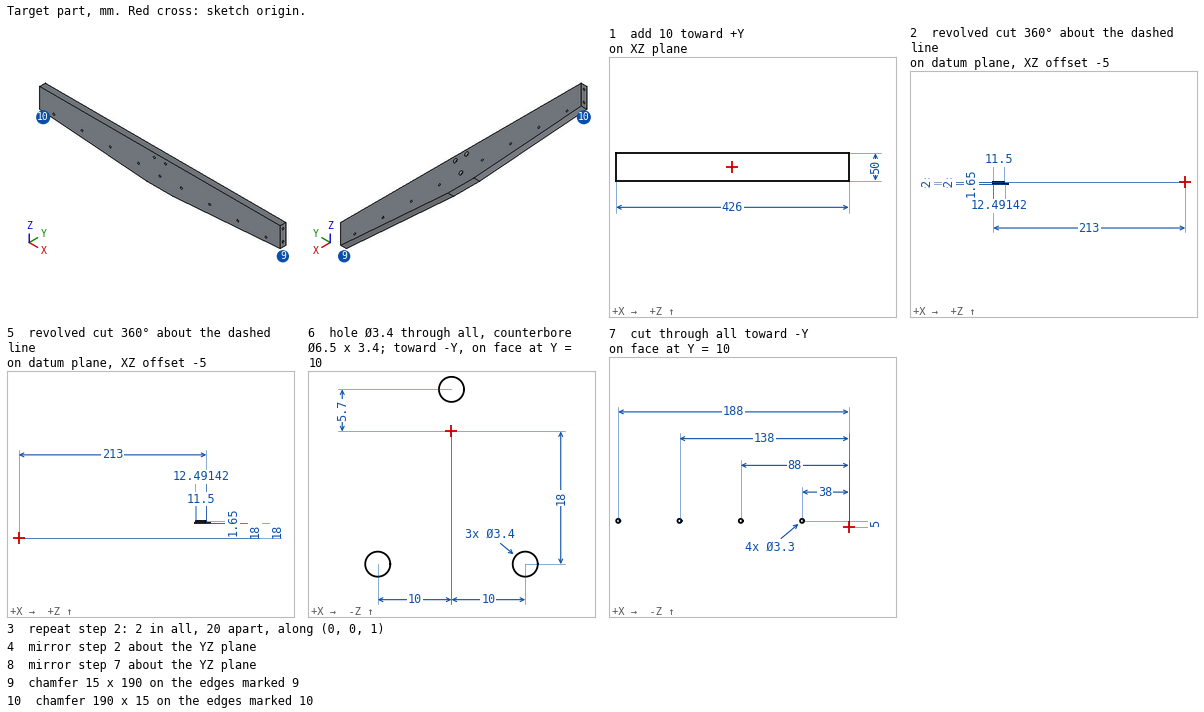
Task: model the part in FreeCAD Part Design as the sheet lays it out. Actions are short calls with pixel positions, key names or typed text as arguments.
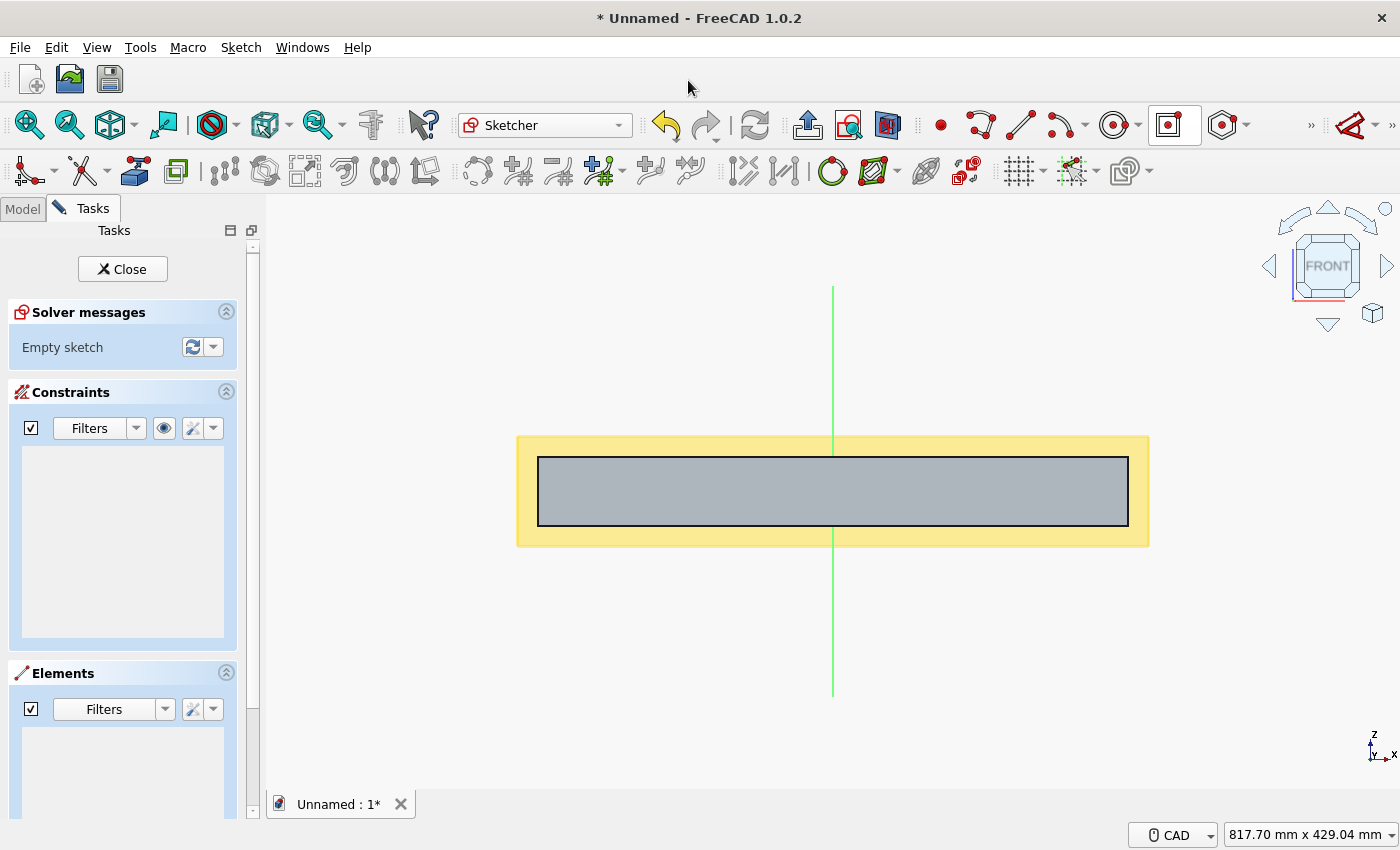
click(888, 126)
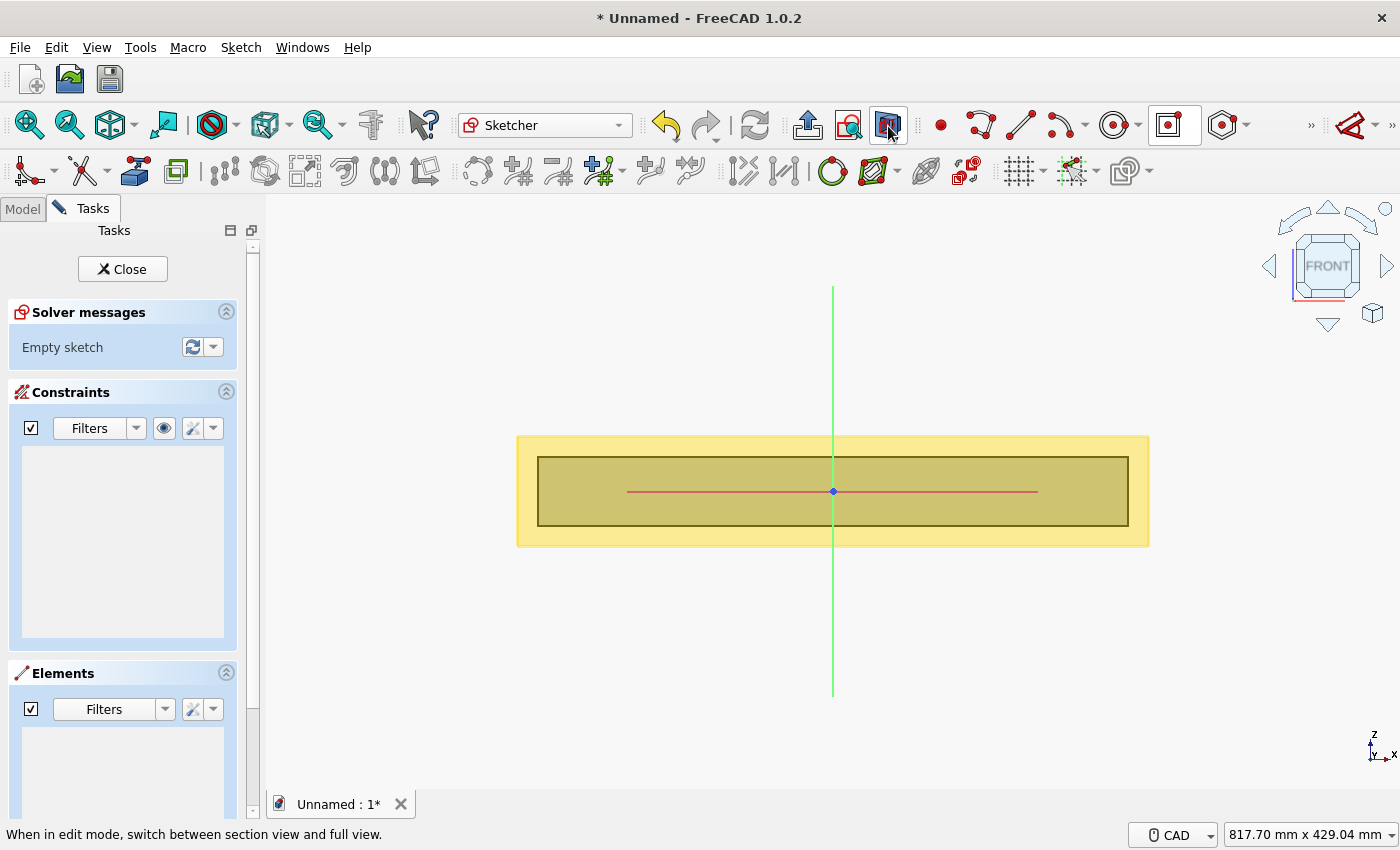
scroll(538, 493, up, 15)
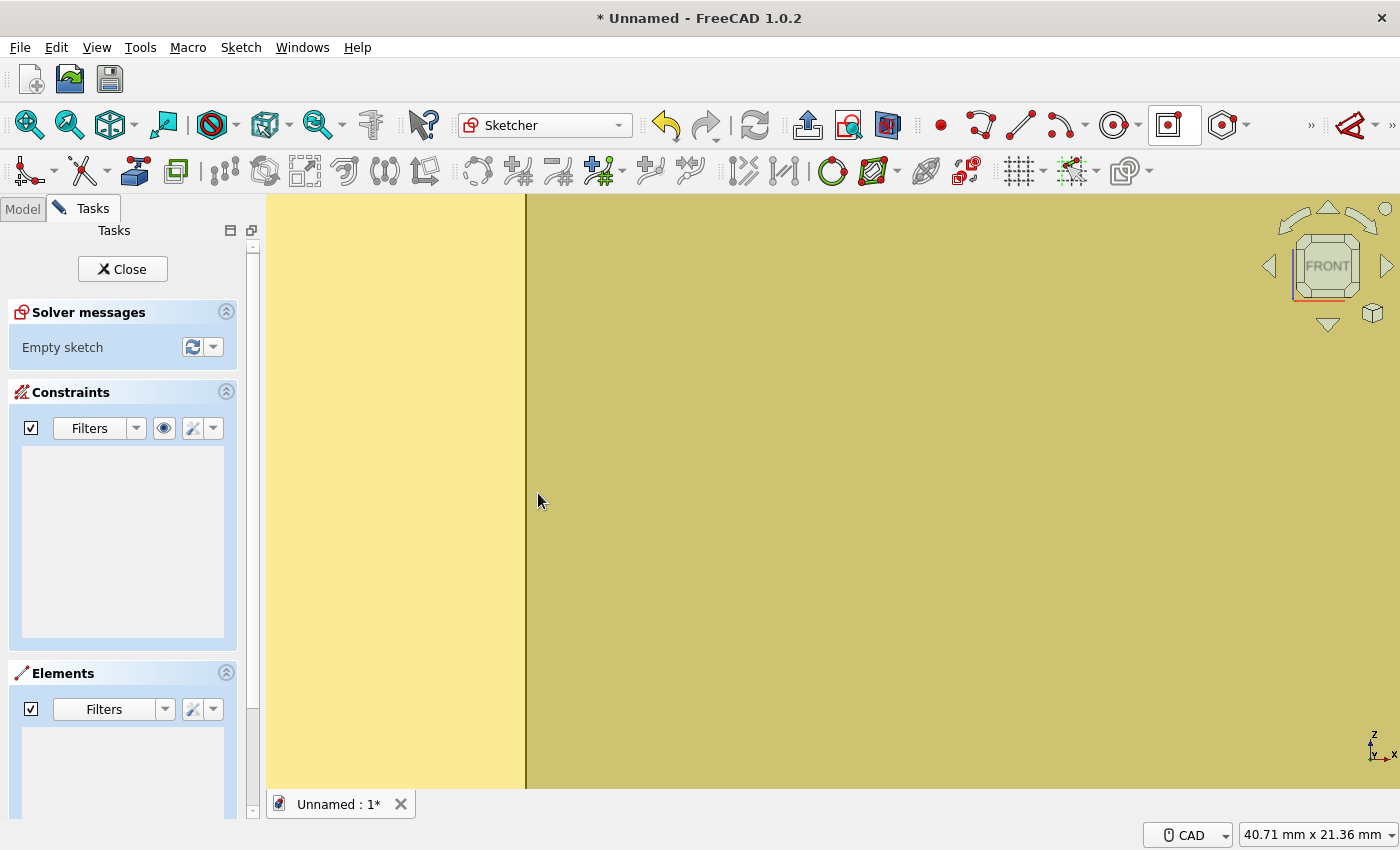
scroll(779, 475, up, 2)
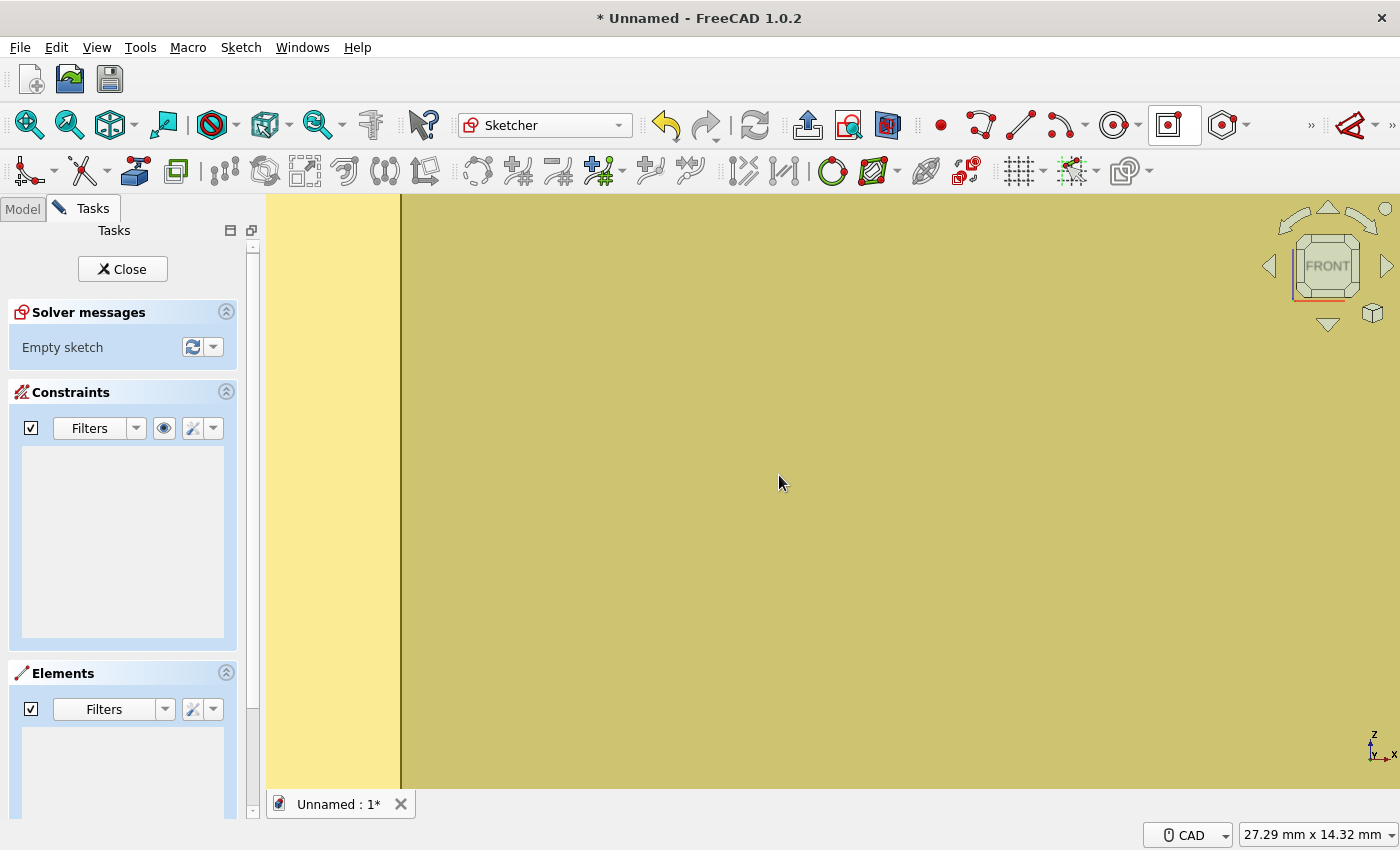
click(982, 126)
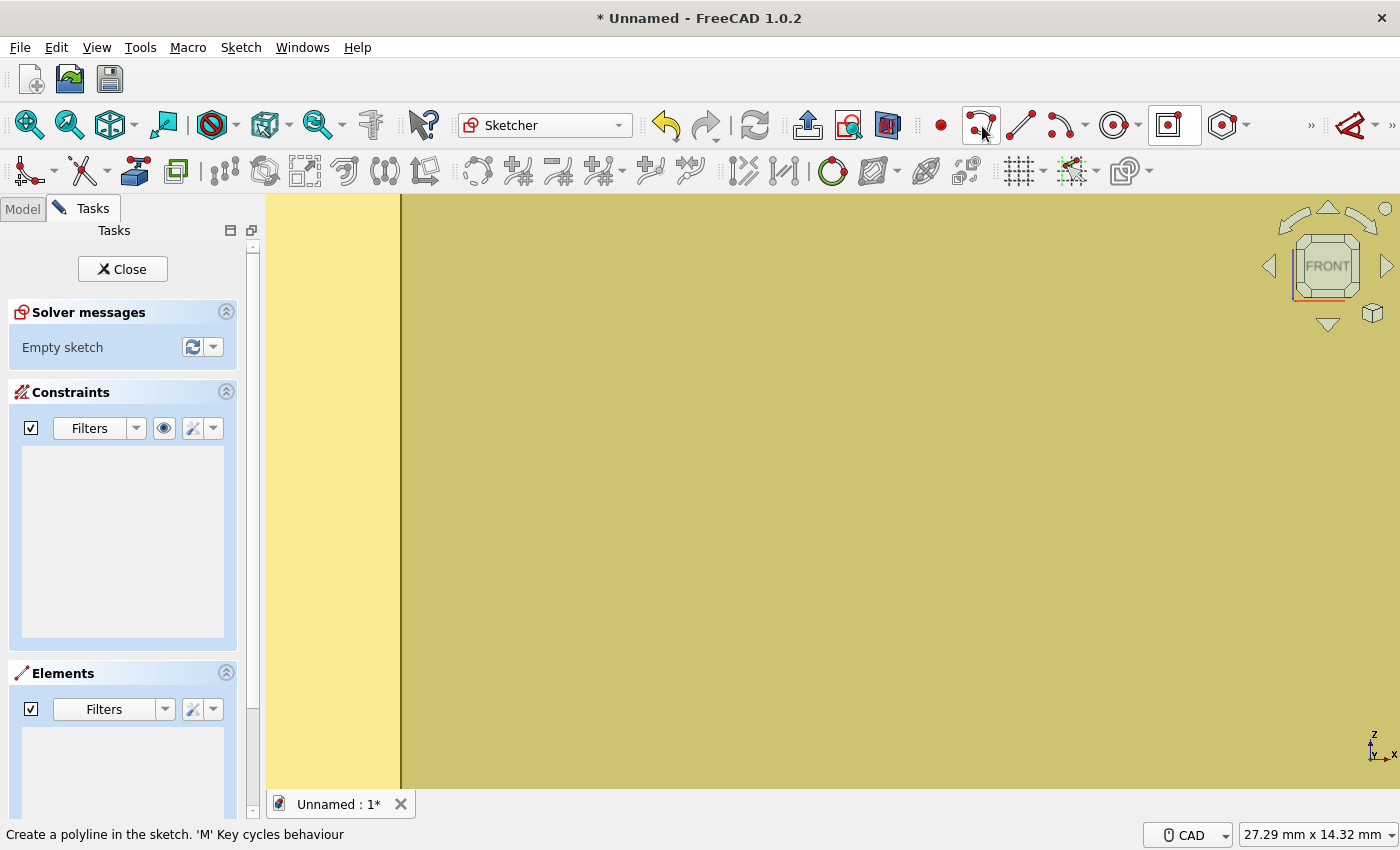
click(920, 525)
click(401, 525)
click(401, 457)
click(879, 457)
click(920, 526)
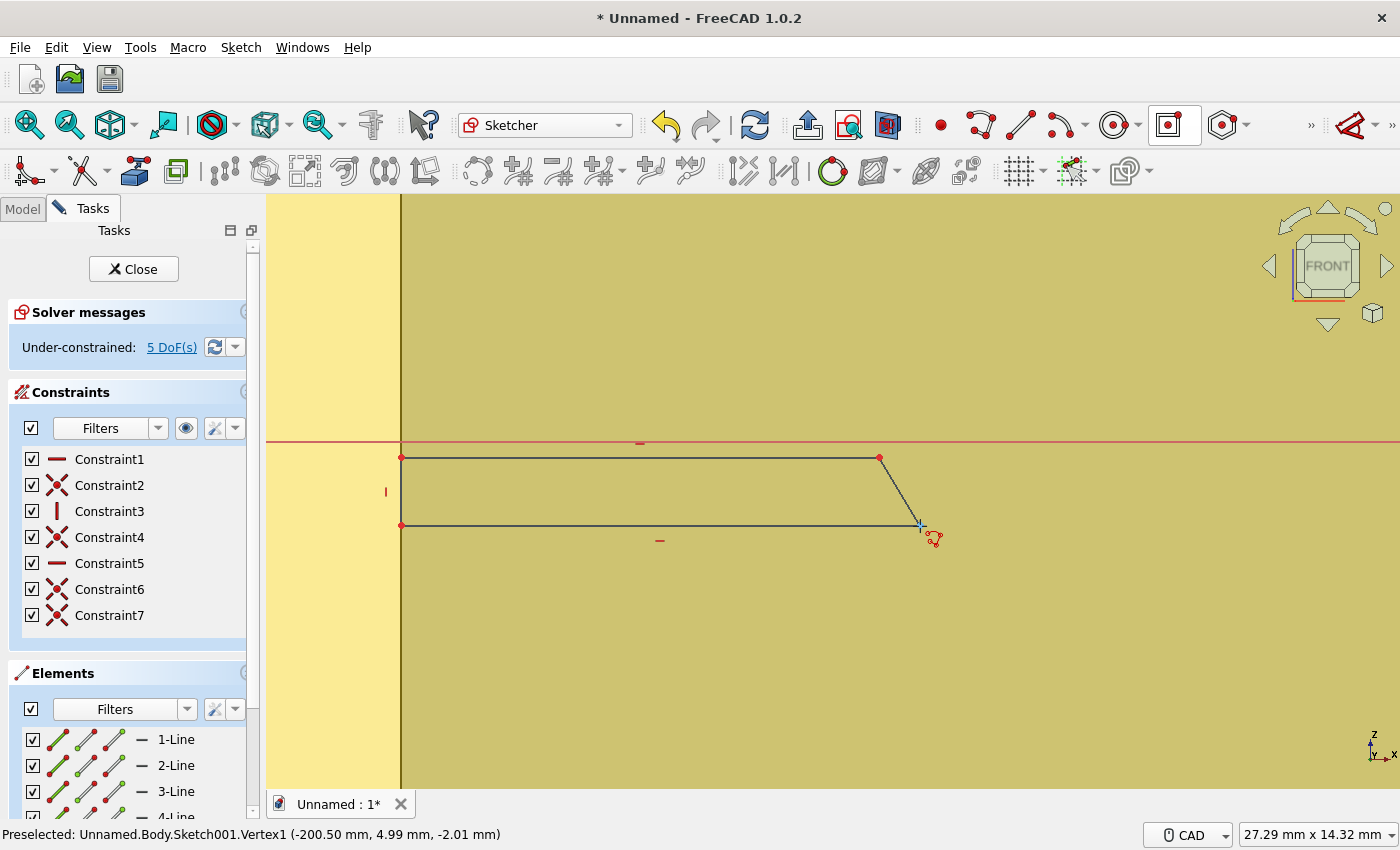
click(1022, 126)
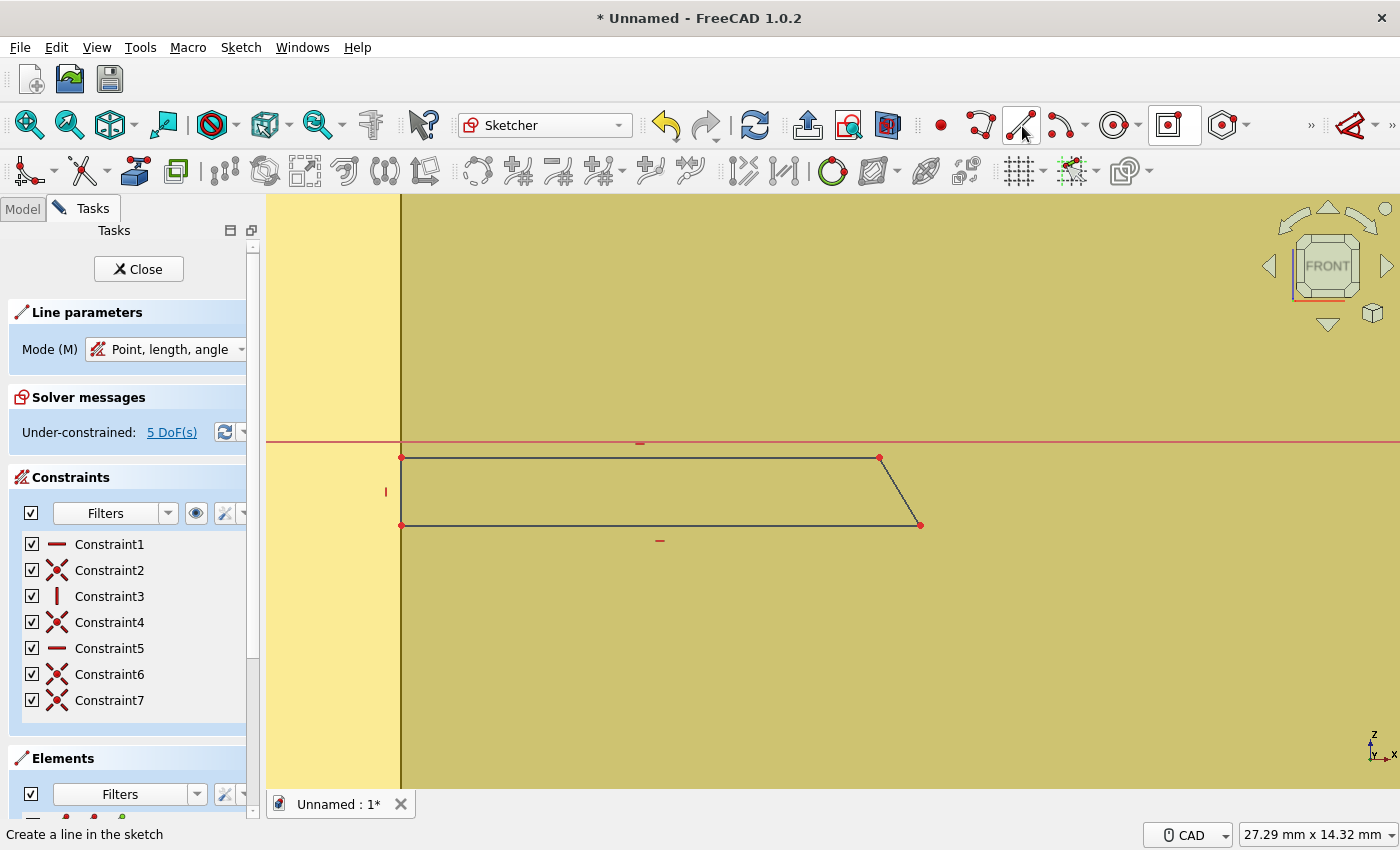
click(972, 525)
click(1127, 525)
key(Escape)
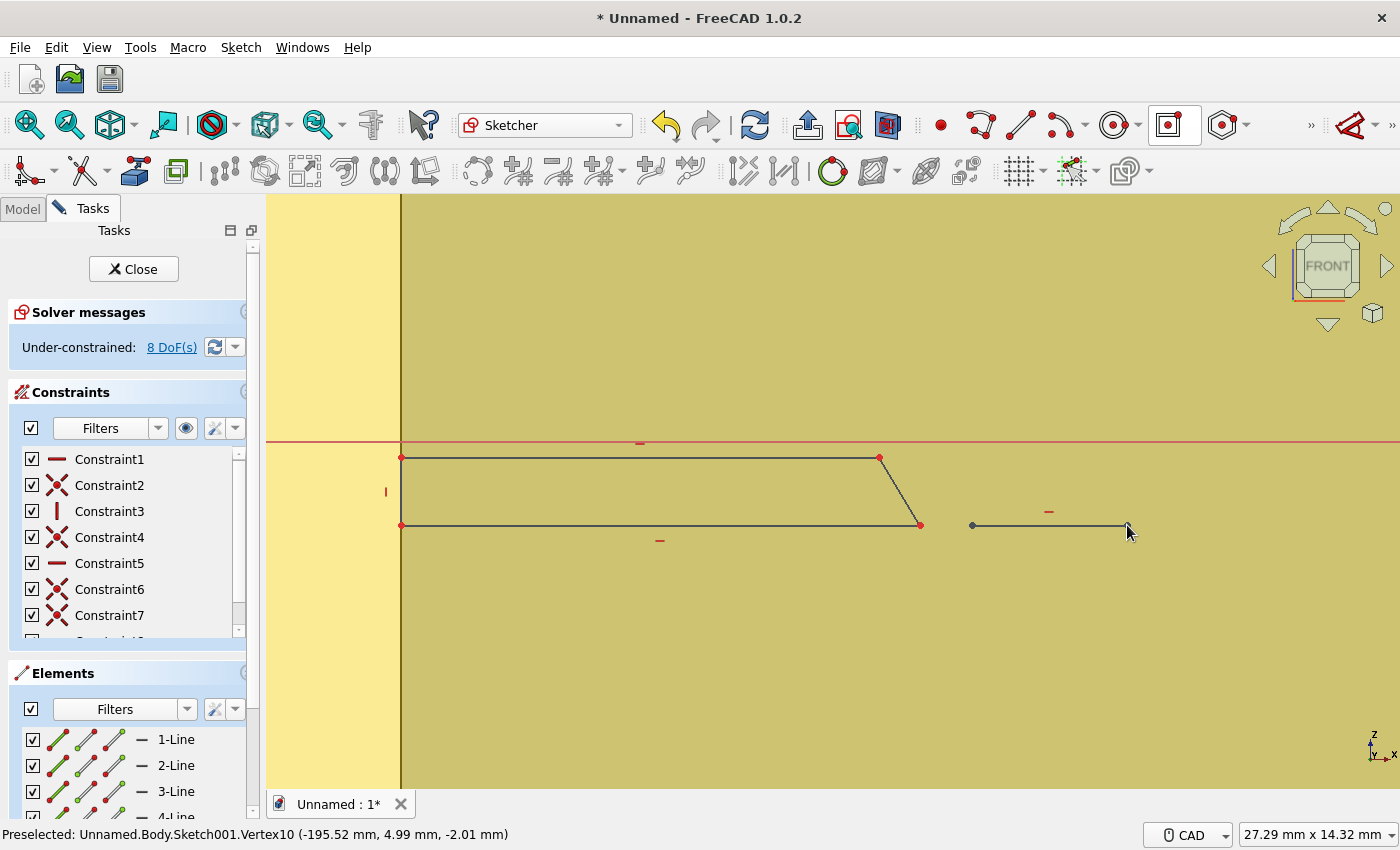
click(1019, 526)